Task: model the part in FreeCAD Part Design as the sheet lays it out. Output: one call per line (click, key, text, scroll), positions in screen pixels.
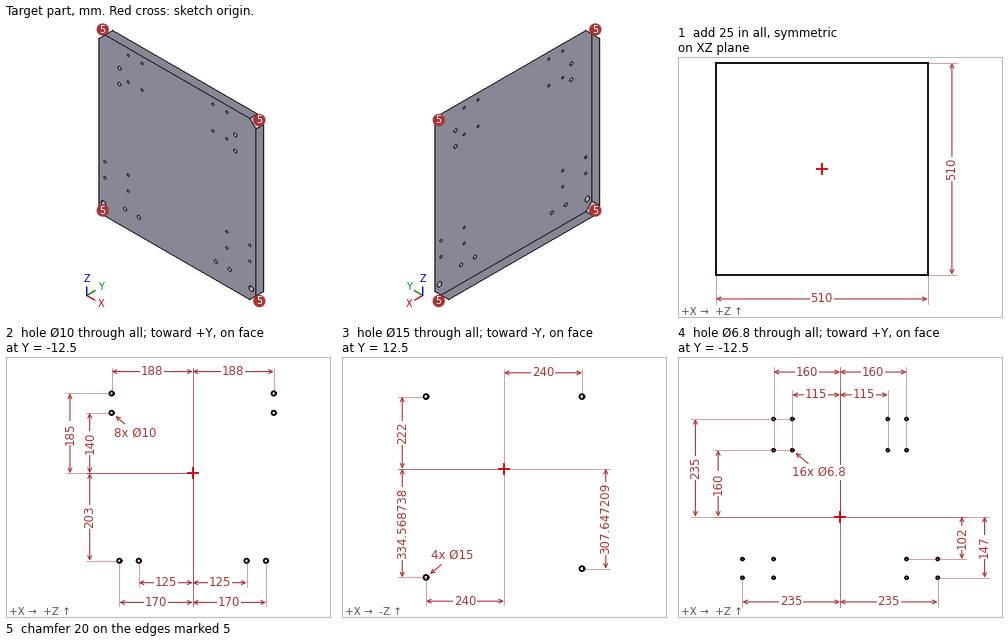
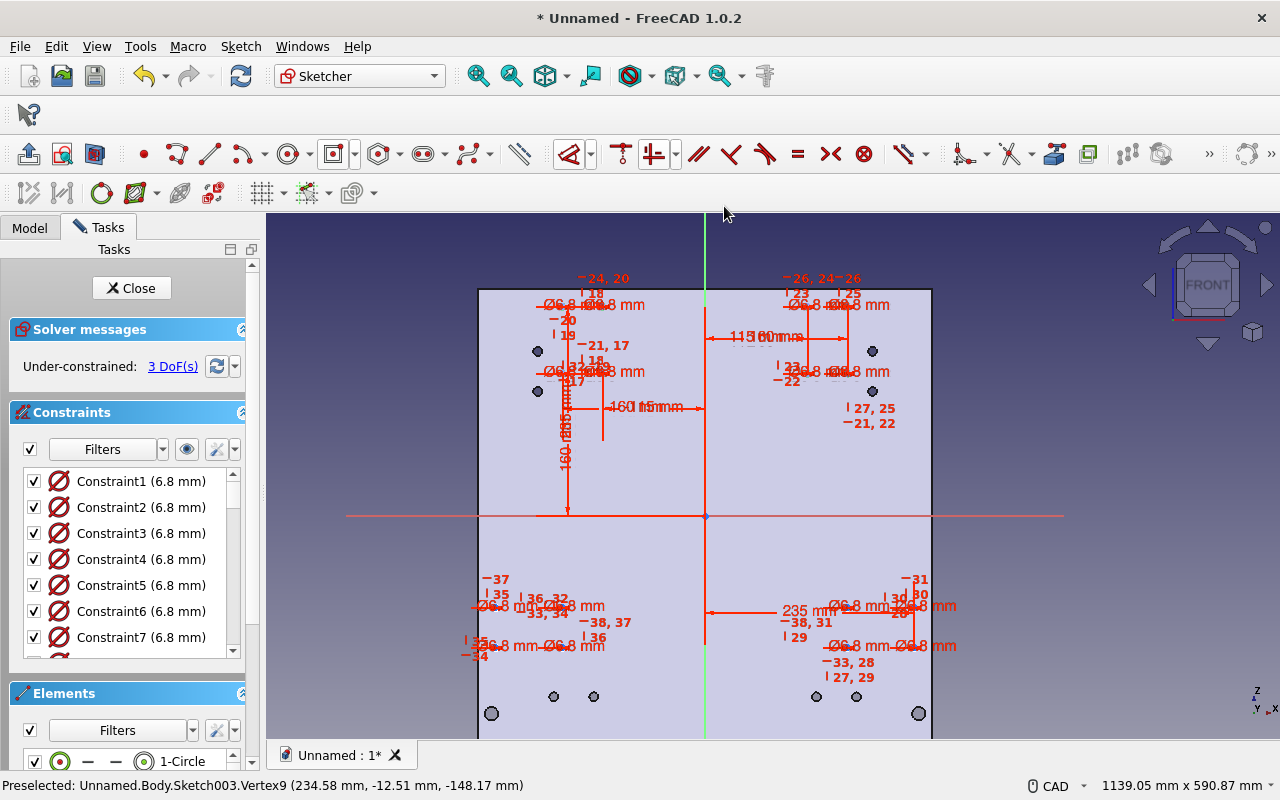
click(914, 648)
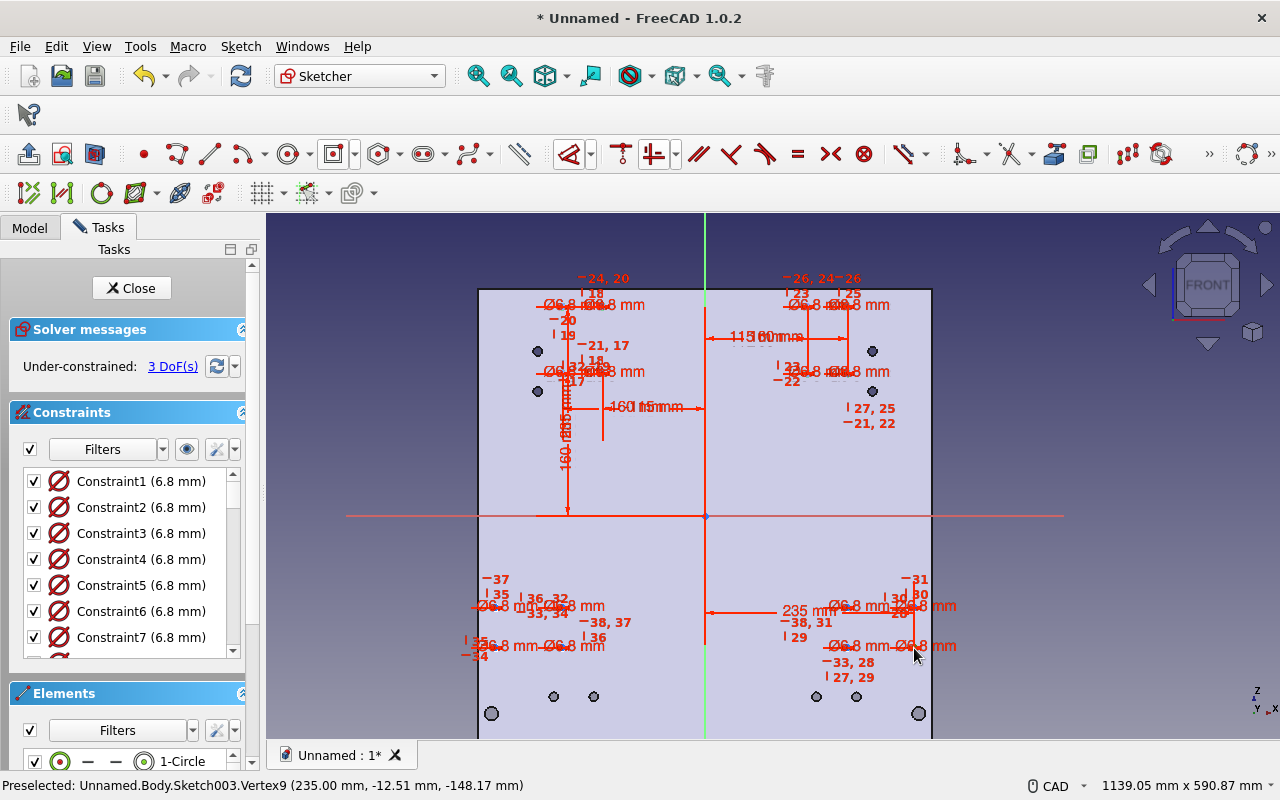
key(i)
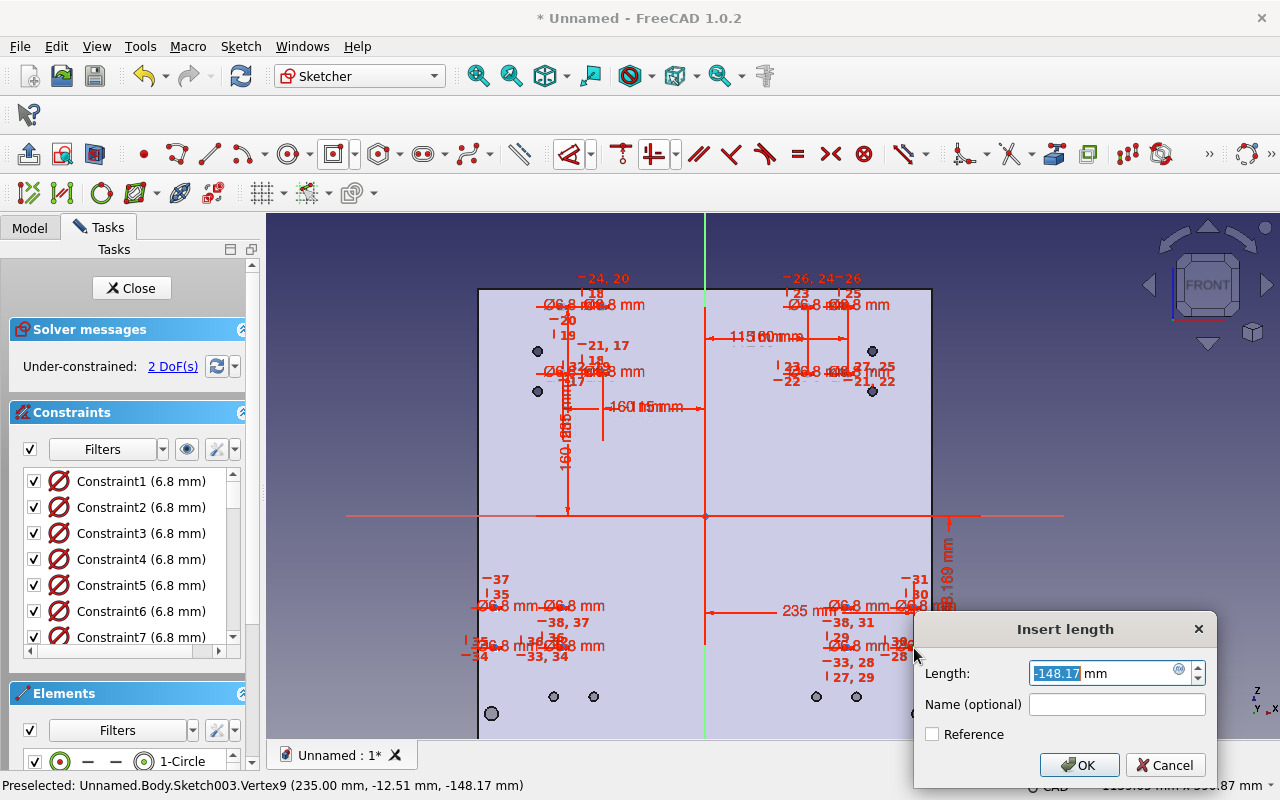
text(-147)
key(Return)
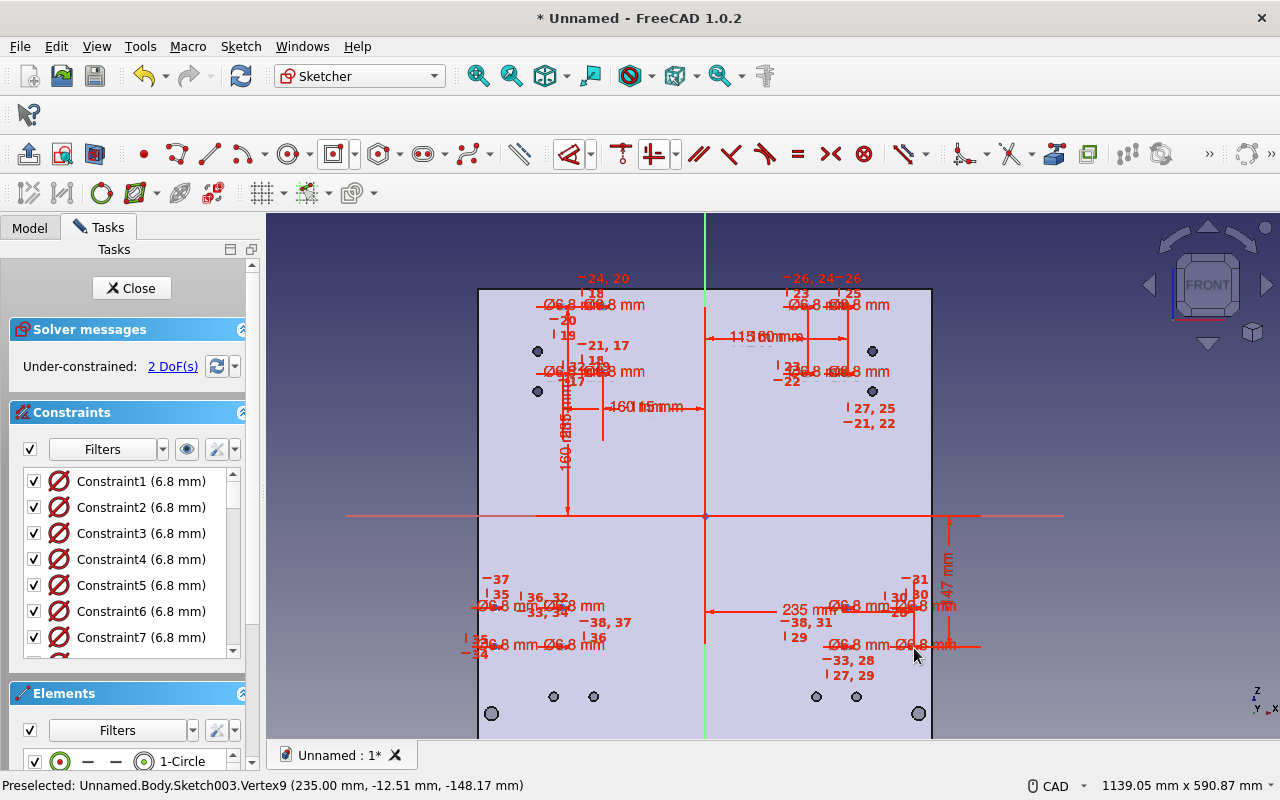
click(848, 608)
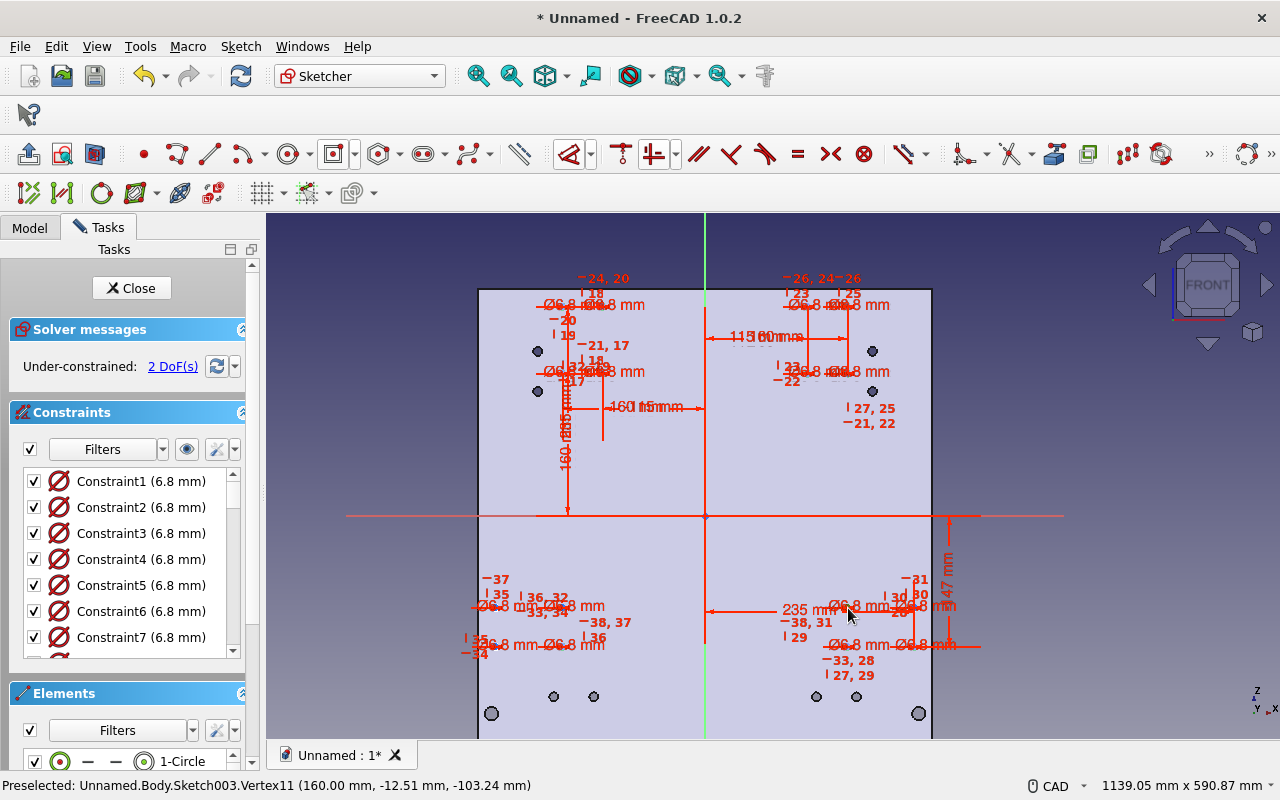
click(590, 154)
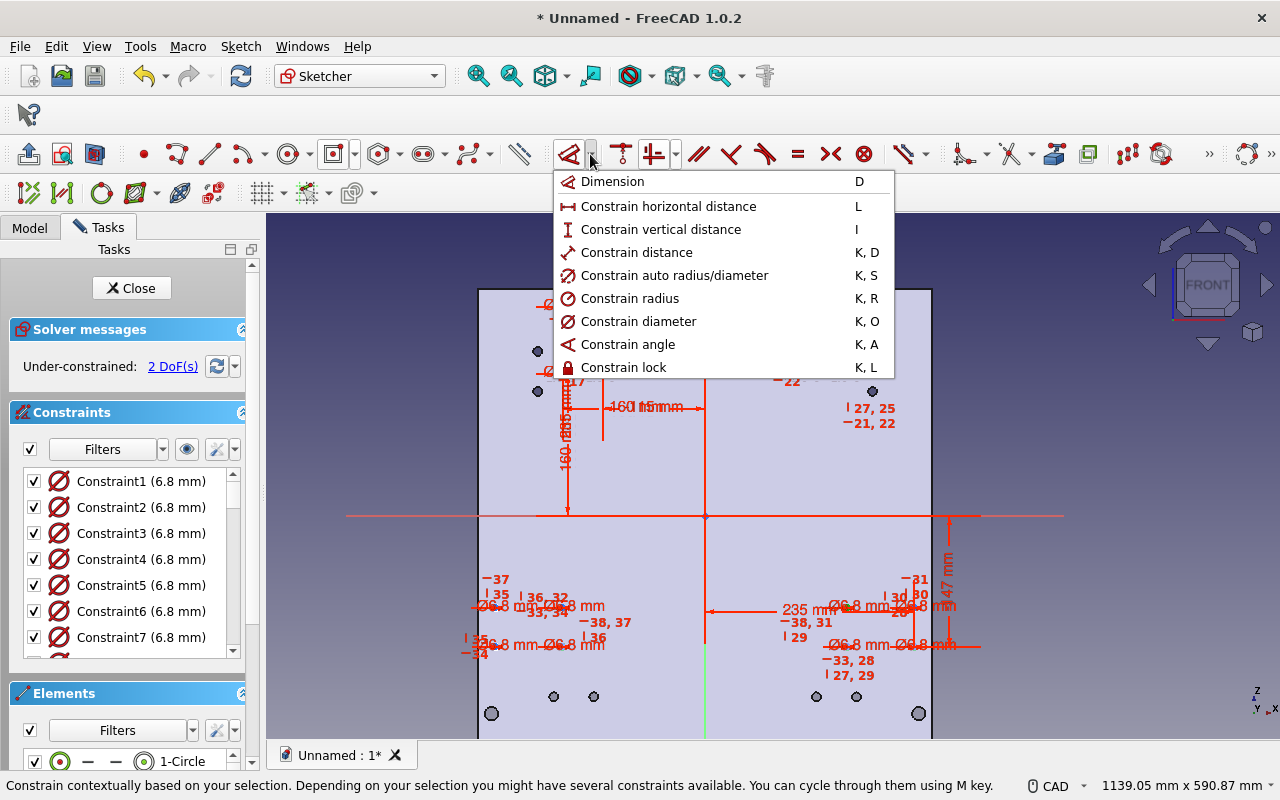
click(724, 230)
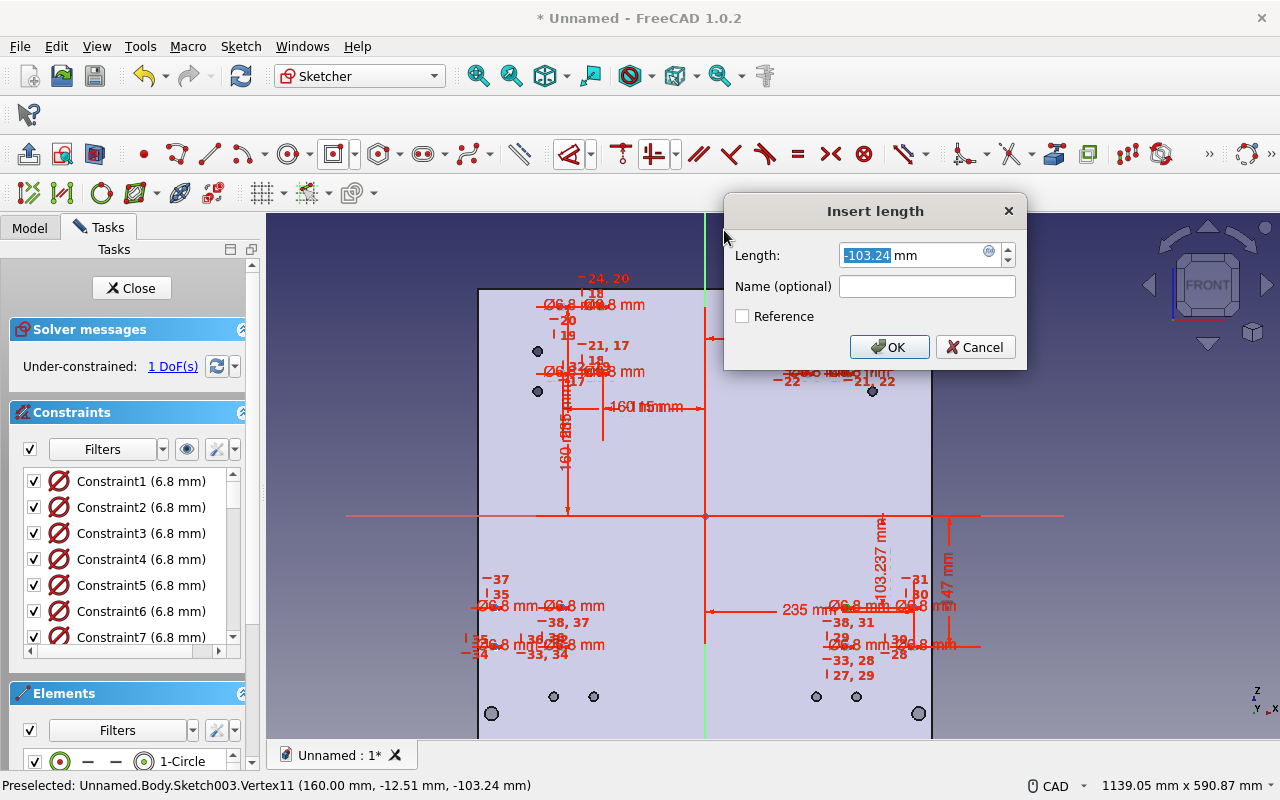
text(-102)
key(Return)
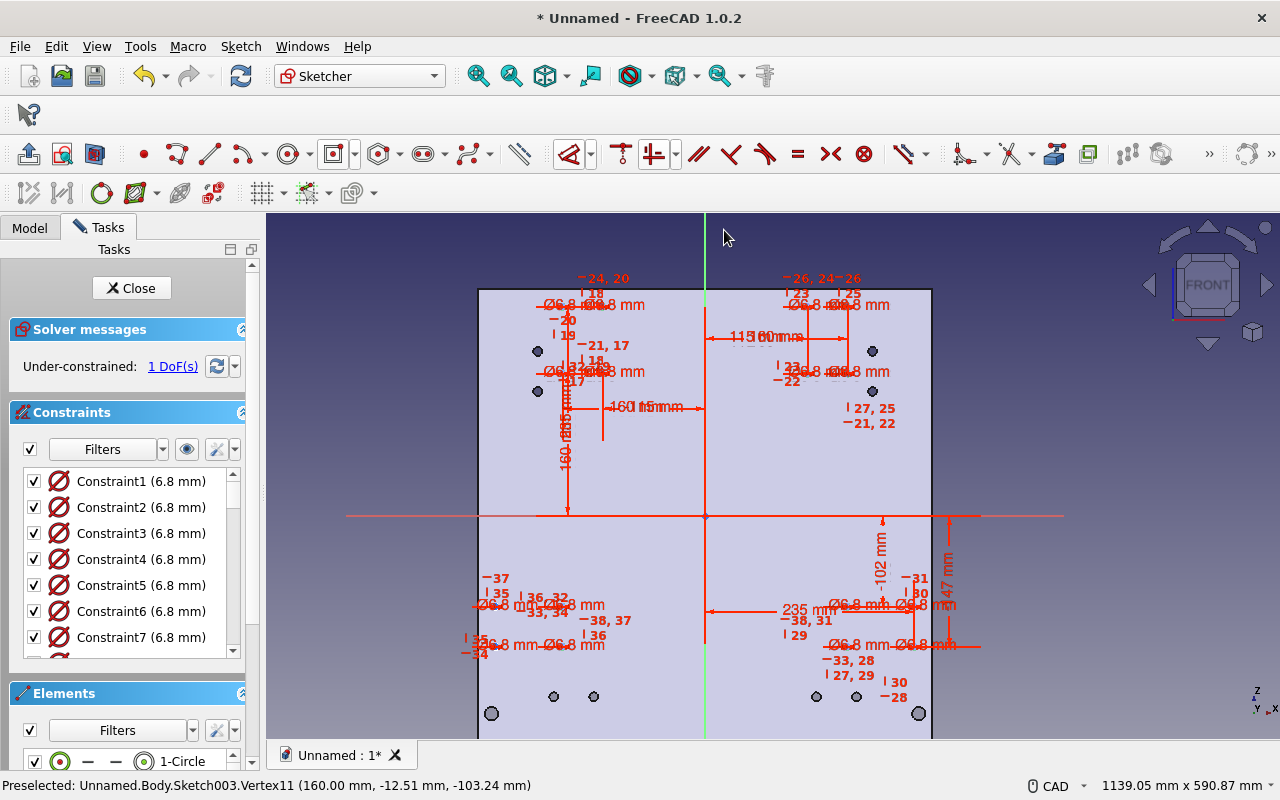
click(496, 647)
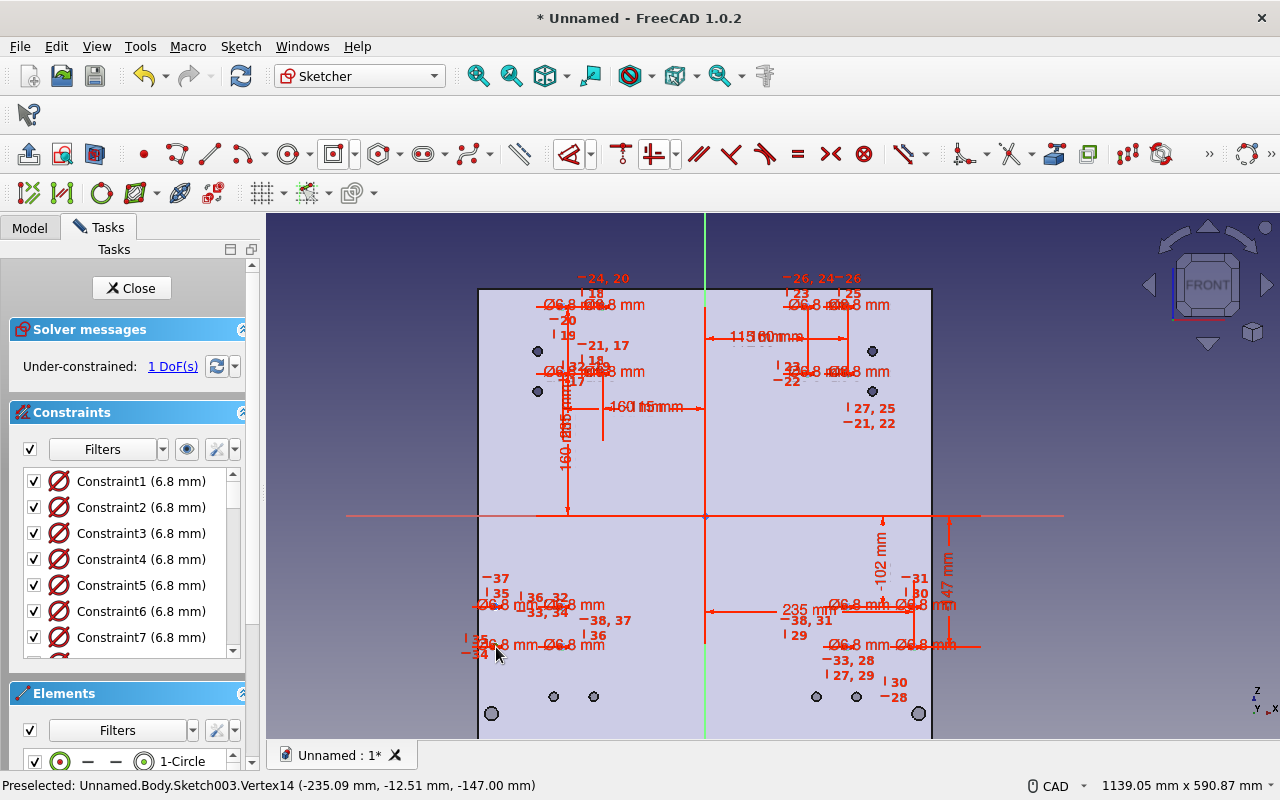
key(l)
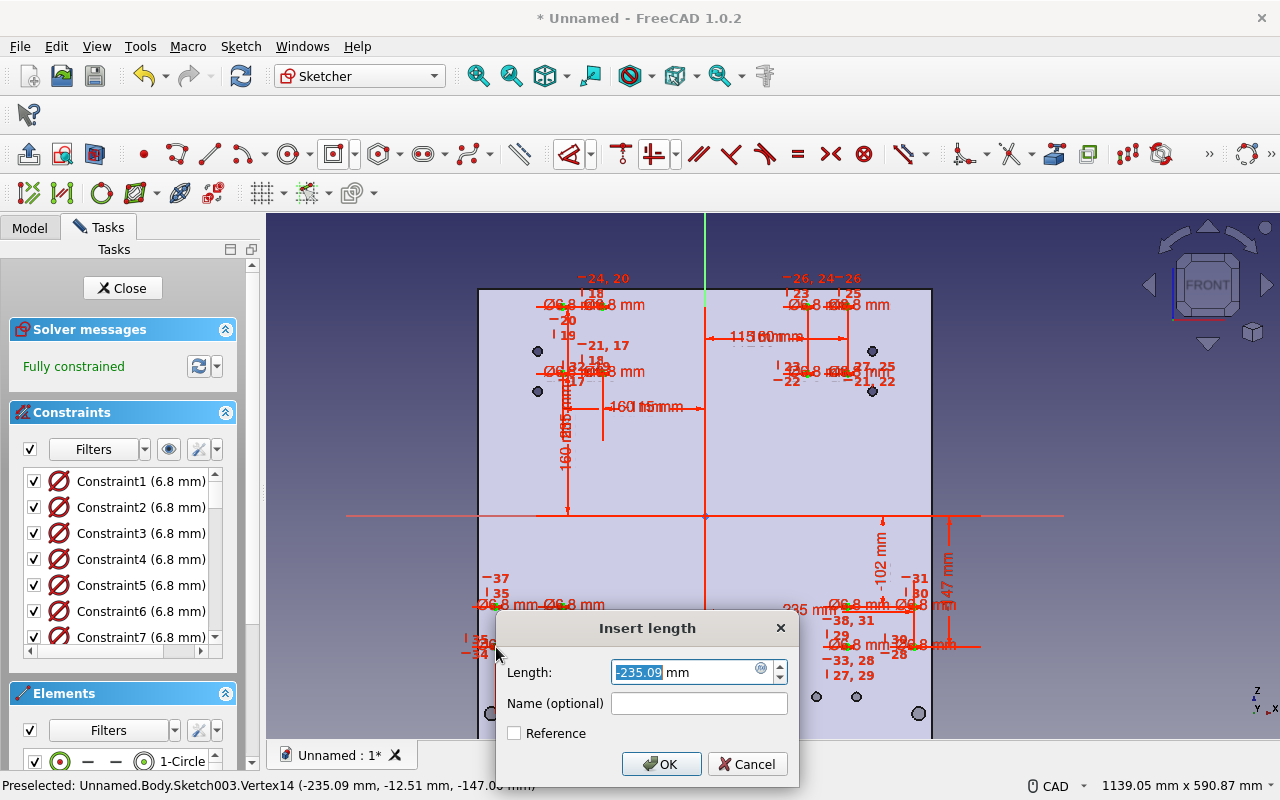
text(-235)
key(Return)